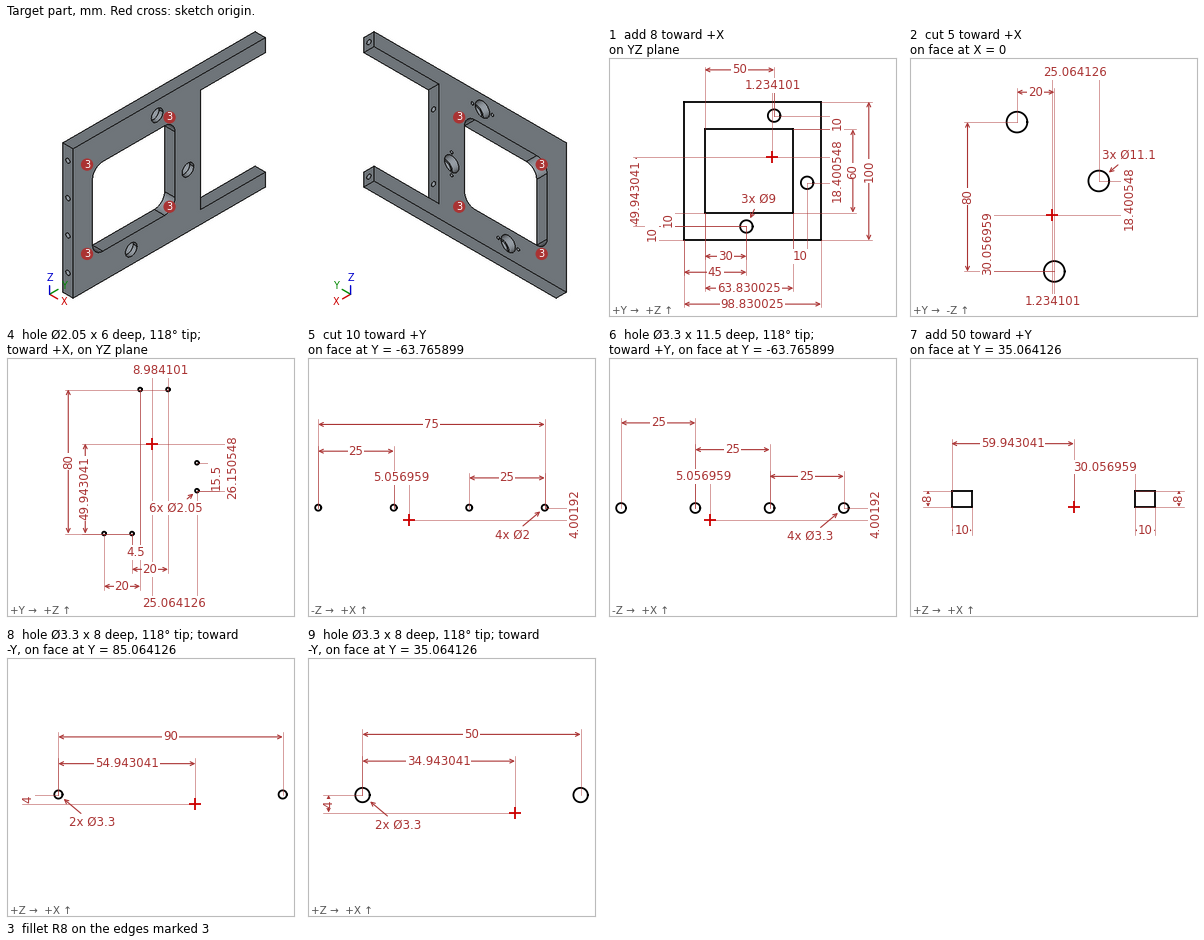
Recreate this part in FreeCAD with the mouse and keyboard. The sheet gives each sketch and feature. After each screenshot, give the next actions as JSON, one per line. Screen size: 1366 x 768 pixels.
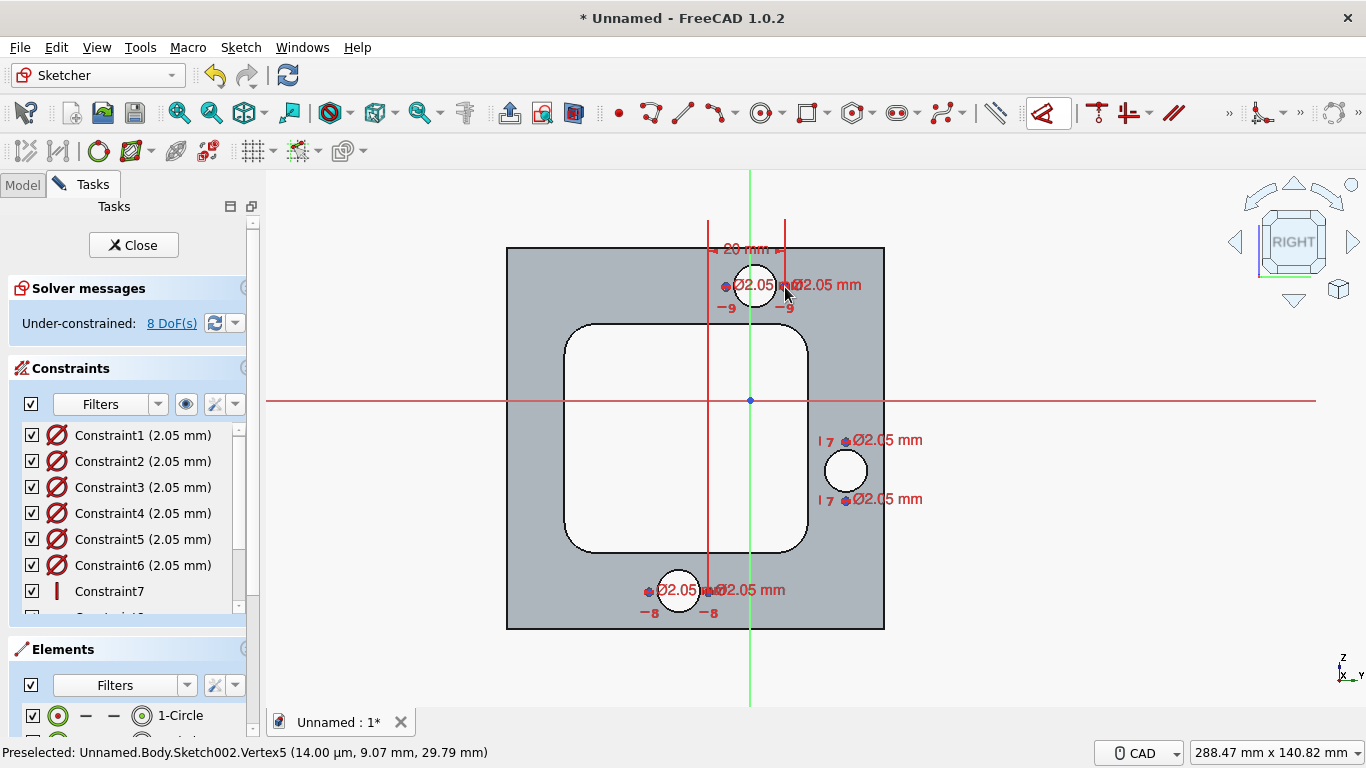
{"action": "left_click", "coordinate": [708, 592]}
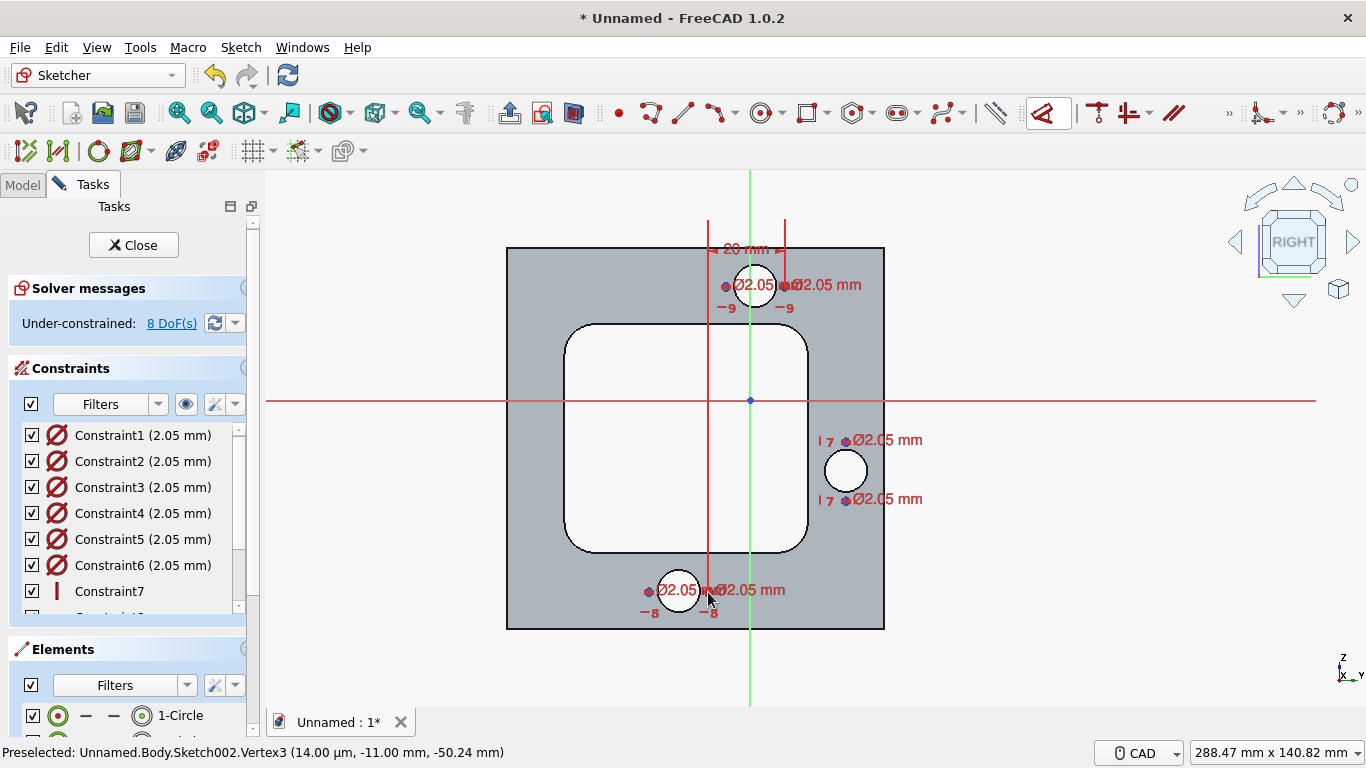
{"action": "left_click", "coordinate": [785, 287]}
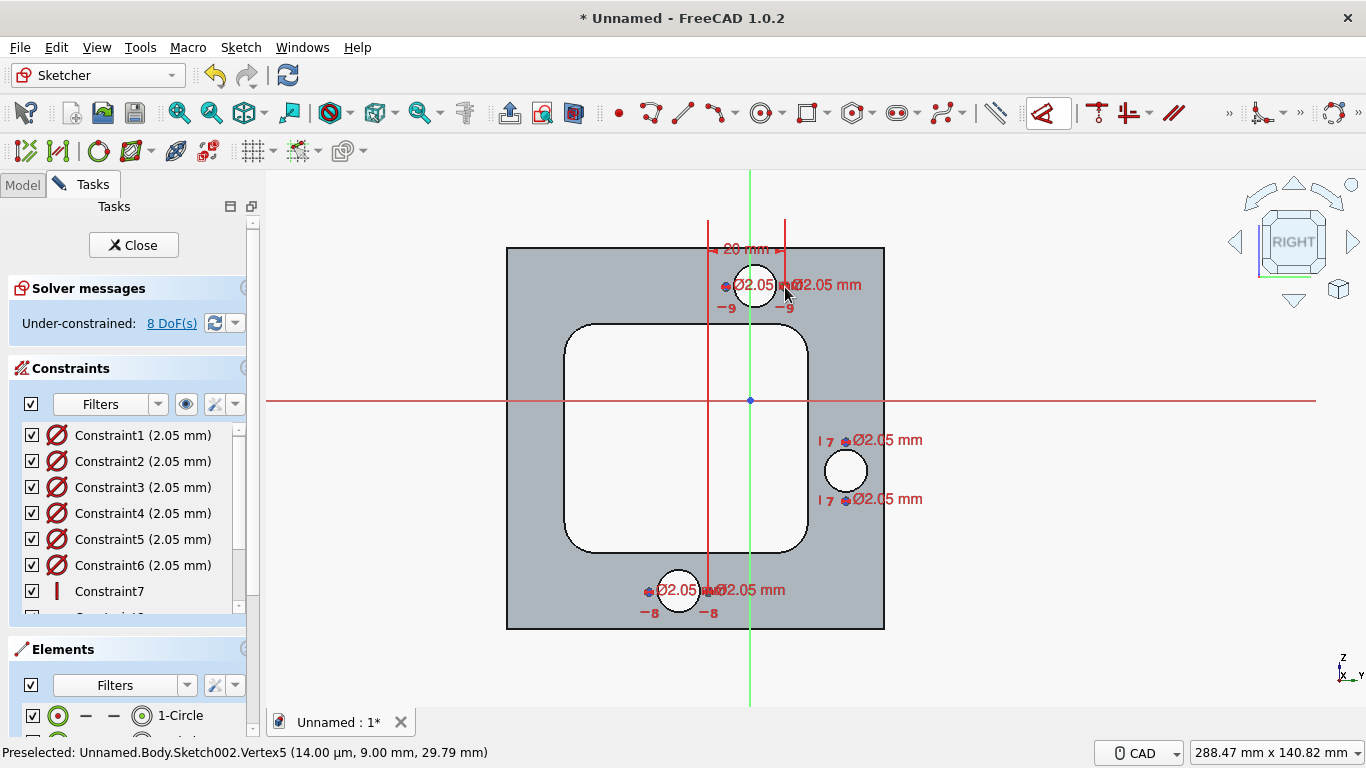
{"action": "key", "text": "i"}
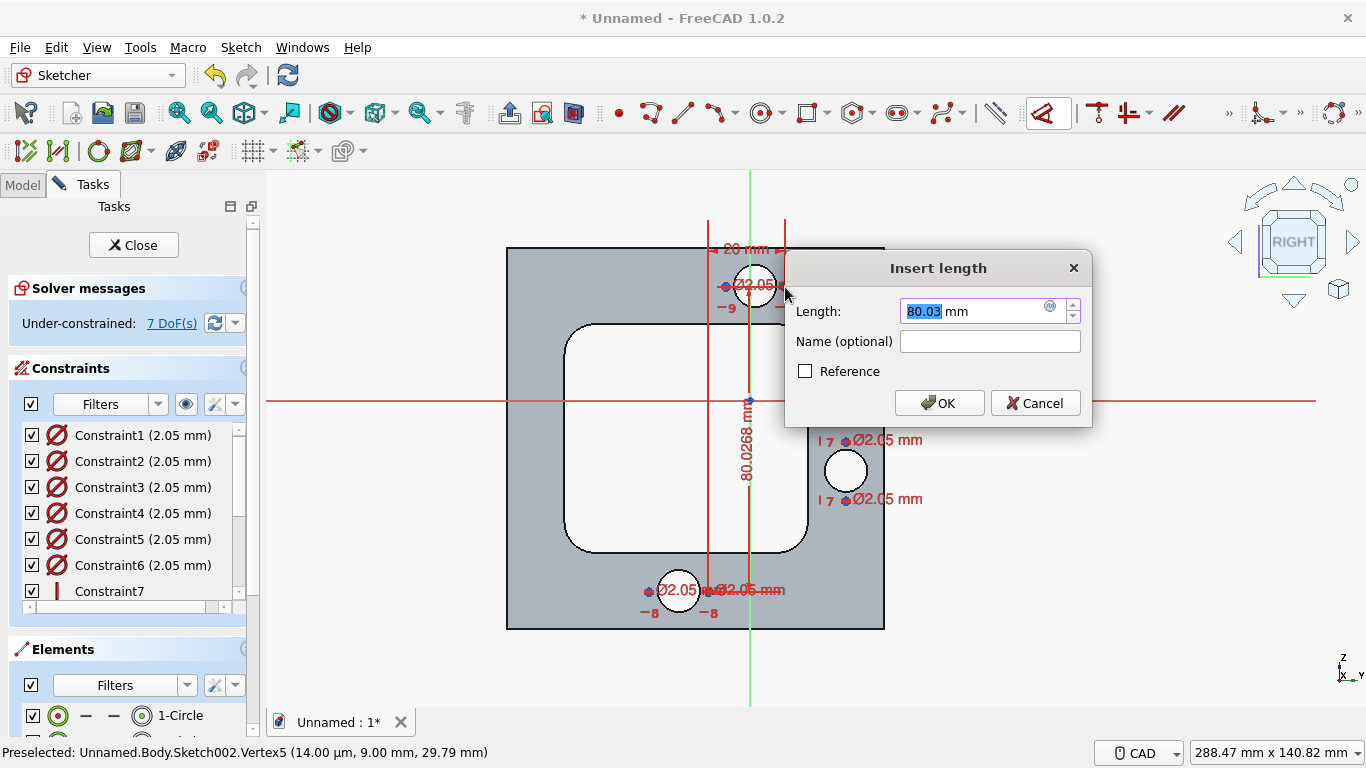
{"action": "type", "text": "80"}
{"action": "key", "text": "Return"}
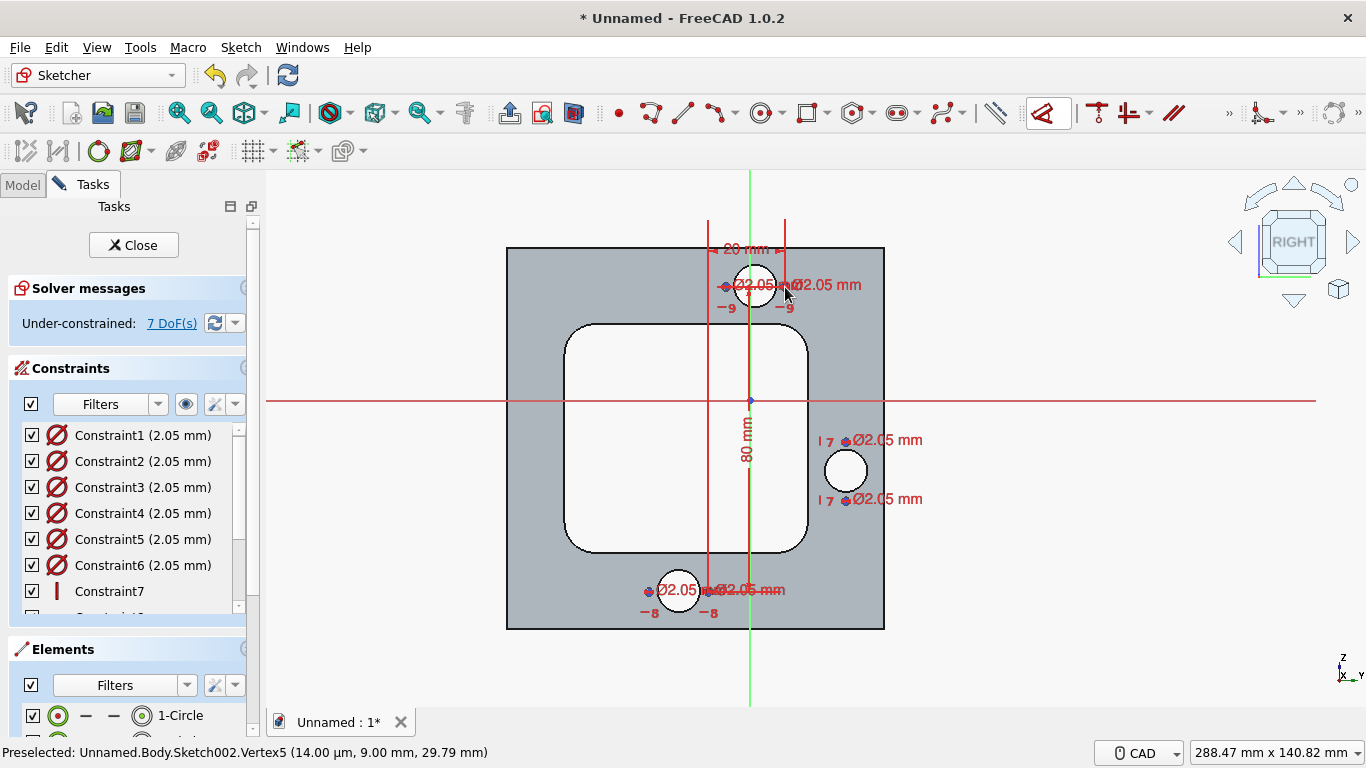
{"action": "left_click", "coordinate": [649, 592]}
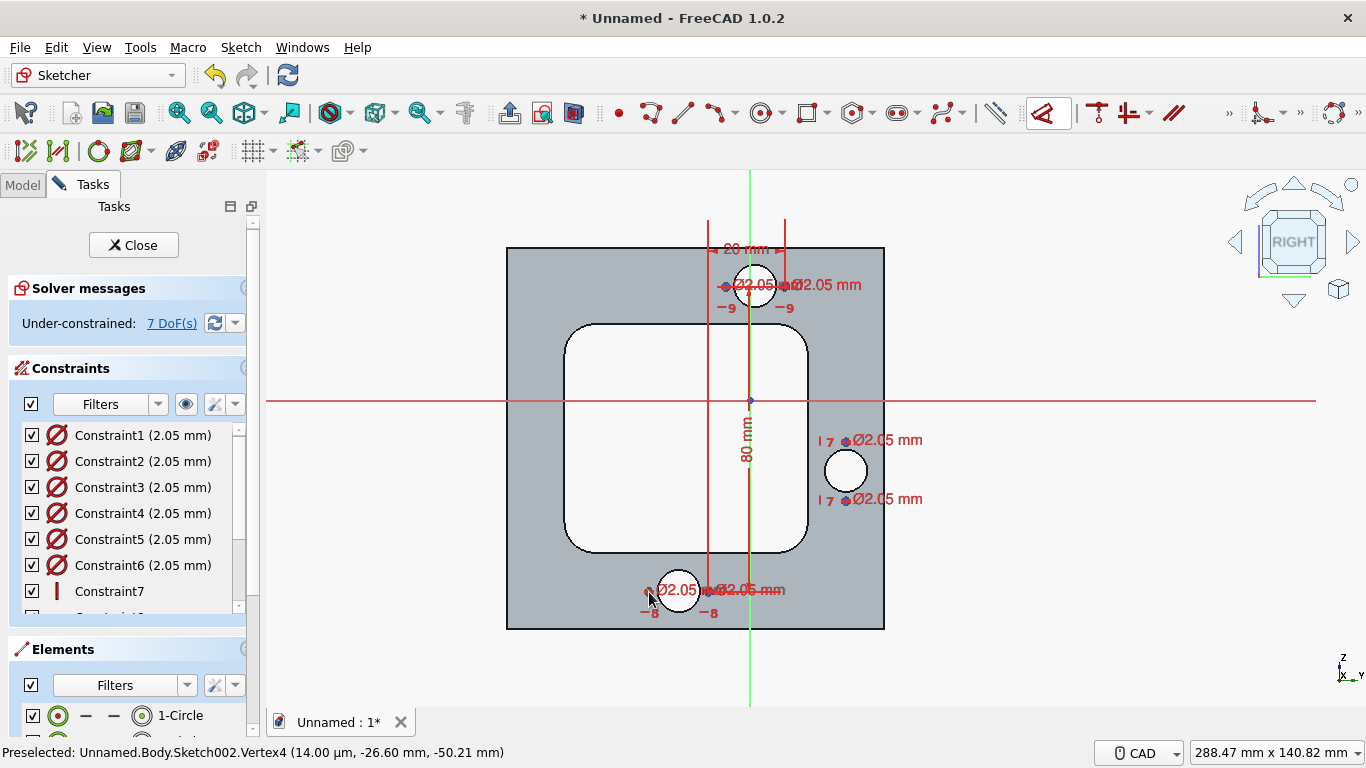
{"action": "left_click", "coordinate": [726, 287]}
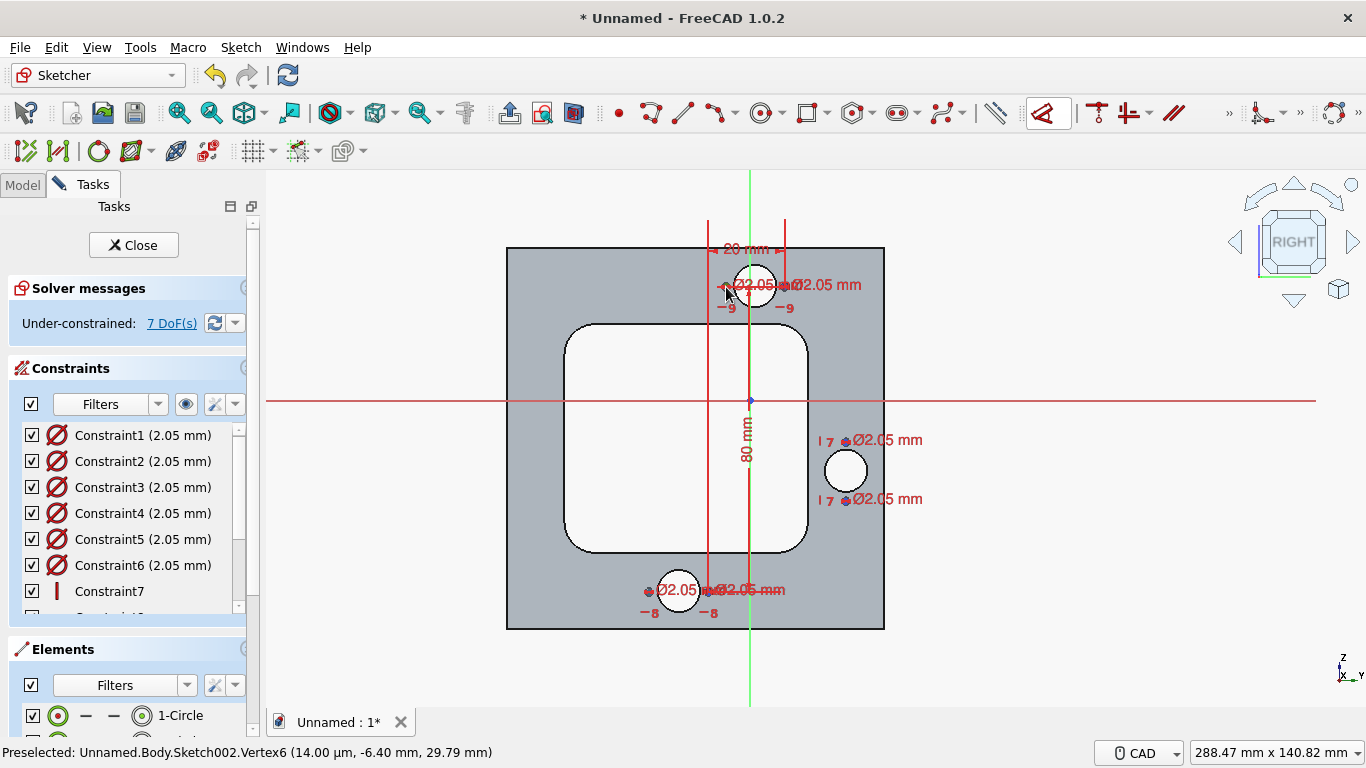
{"action": "left_click", "coordinate": [1066, 114]}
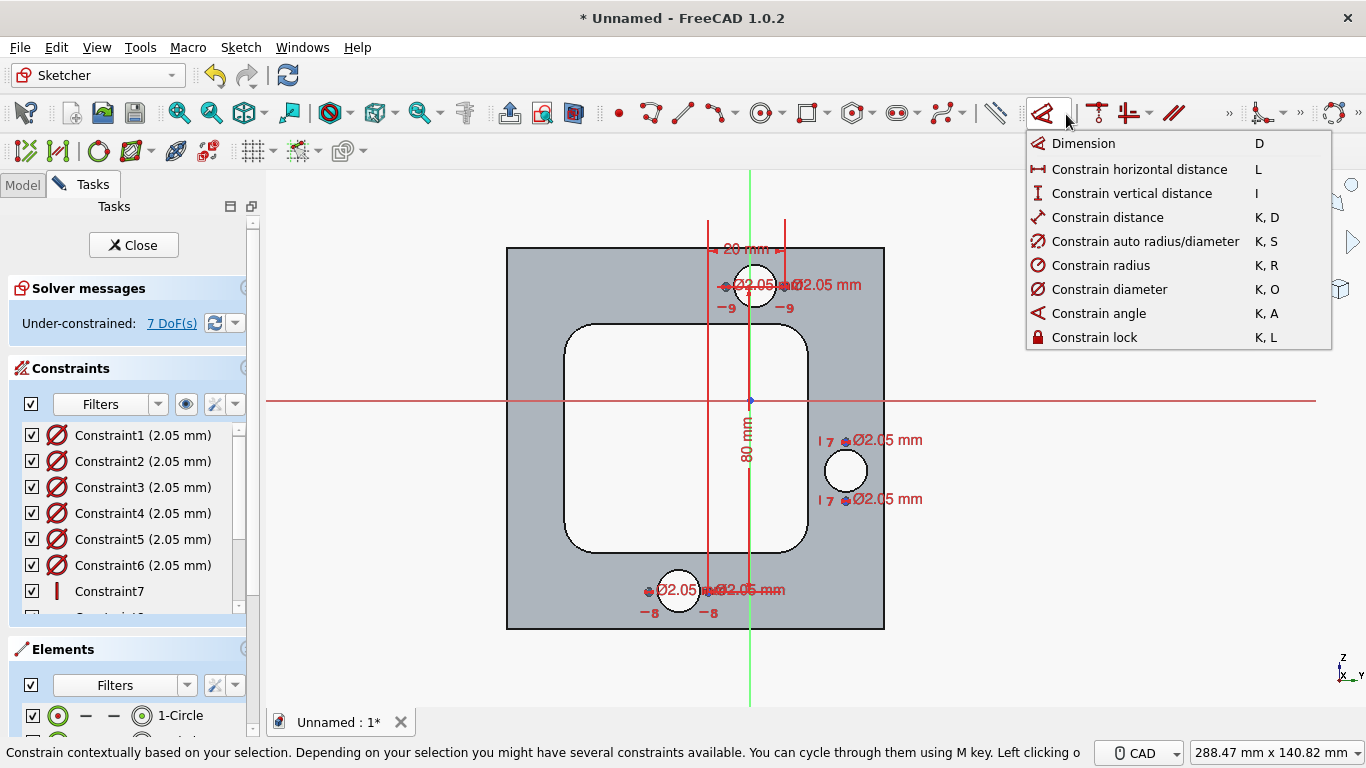
{"action": "left_click", "coordinate": [1179, 169]}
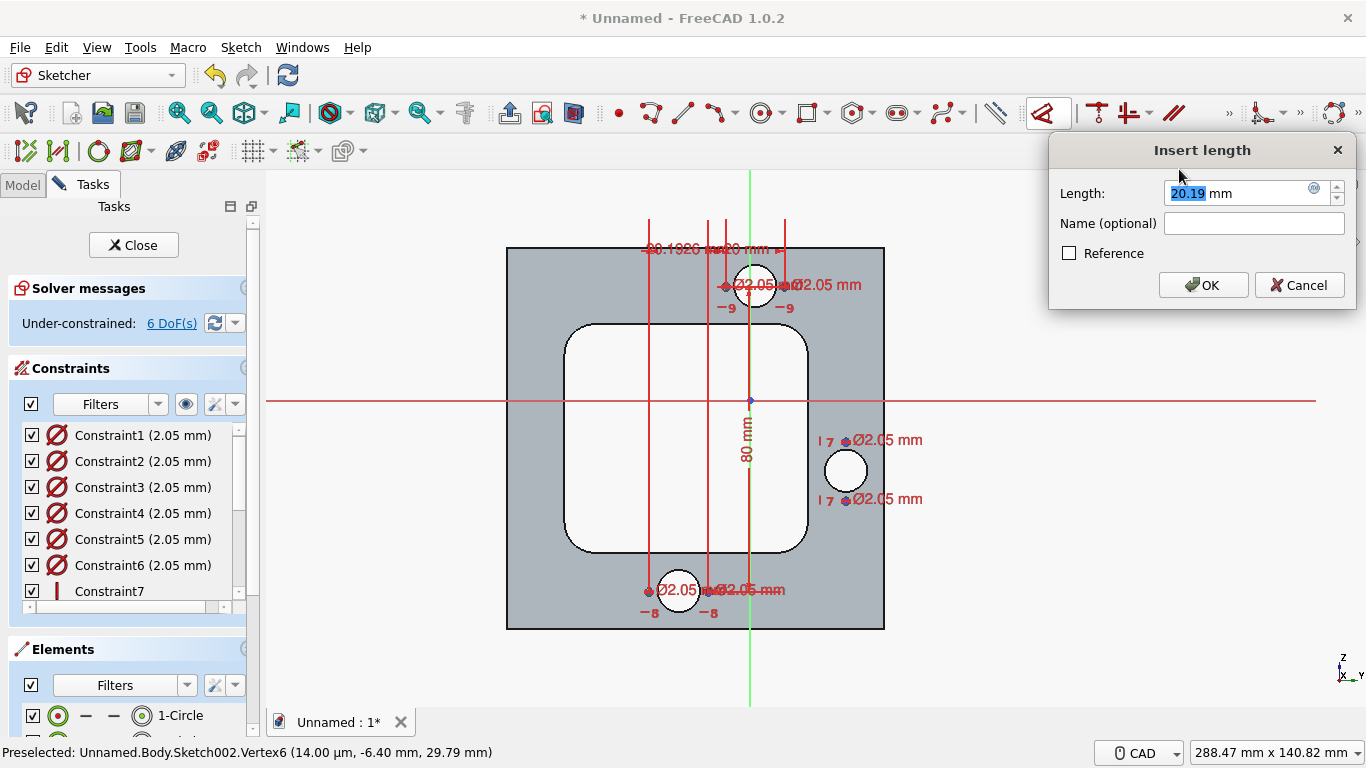
{"action": "type", "text": "20"}
{"action": "key", "text": "Return"}